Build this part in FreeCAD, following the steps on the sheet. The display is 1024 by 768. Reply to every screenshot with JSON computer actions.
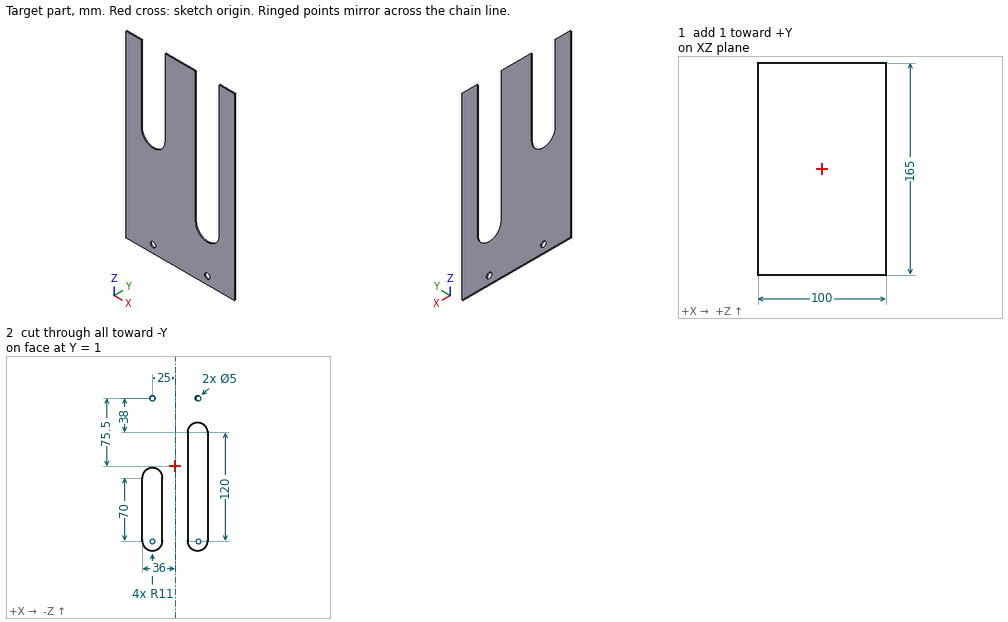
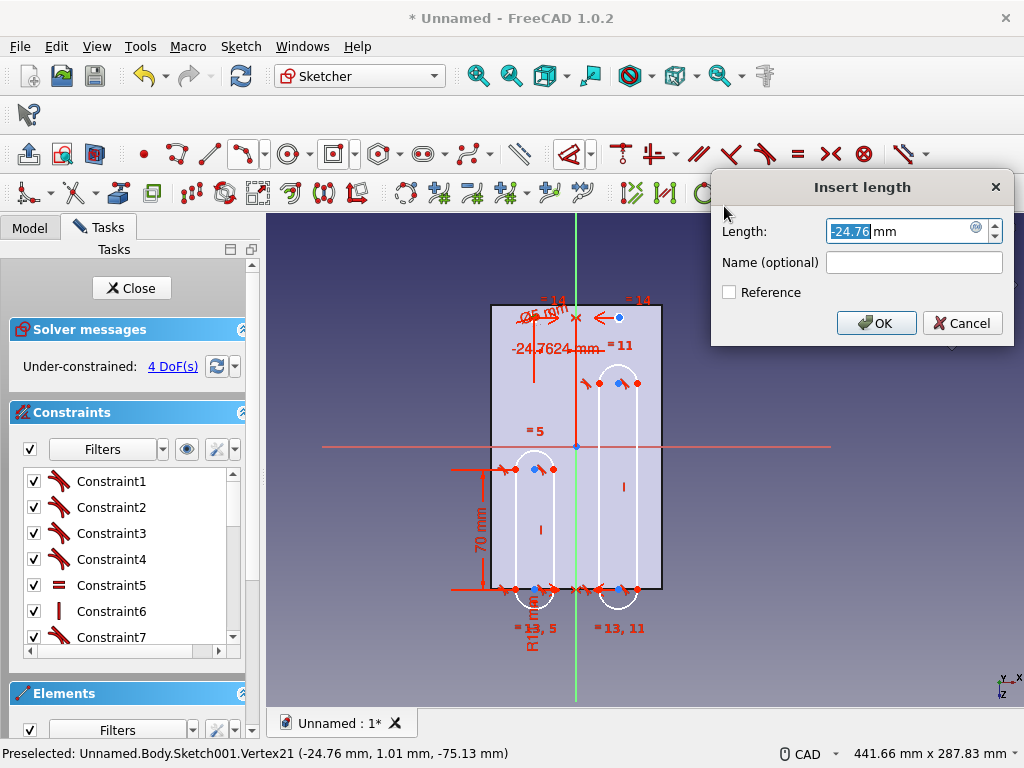
{"action": "type", "text": "-25"}
{"action": "key", "text": "Return"}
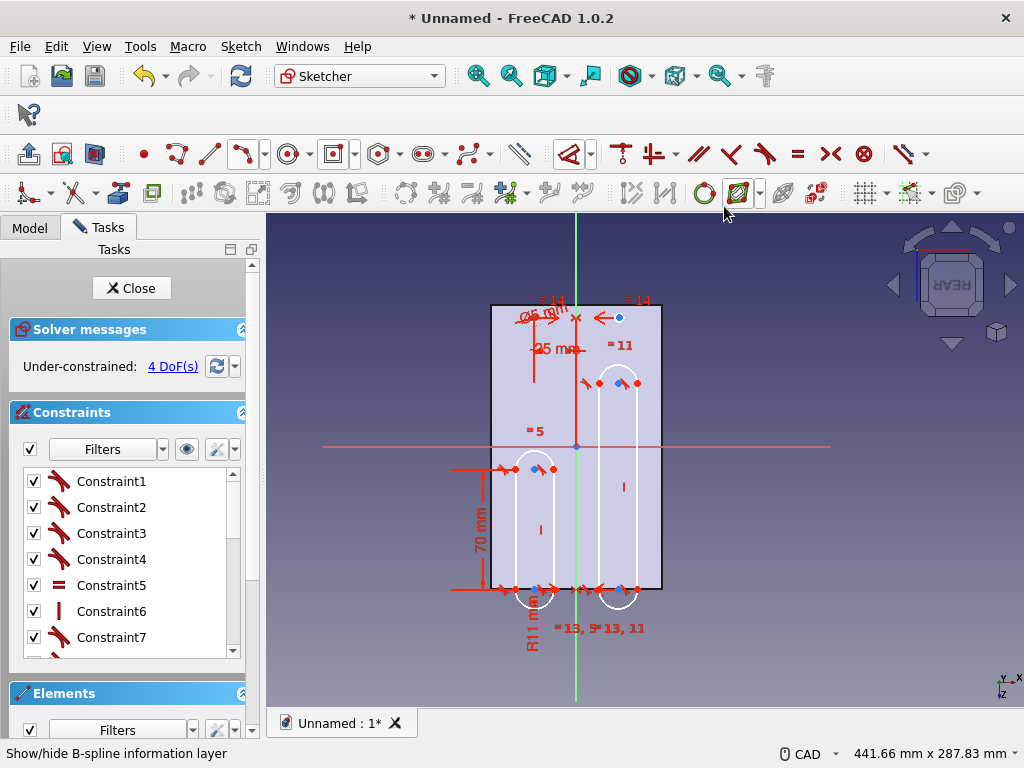
{"action": "left_click", "coordinate": [599, 528]}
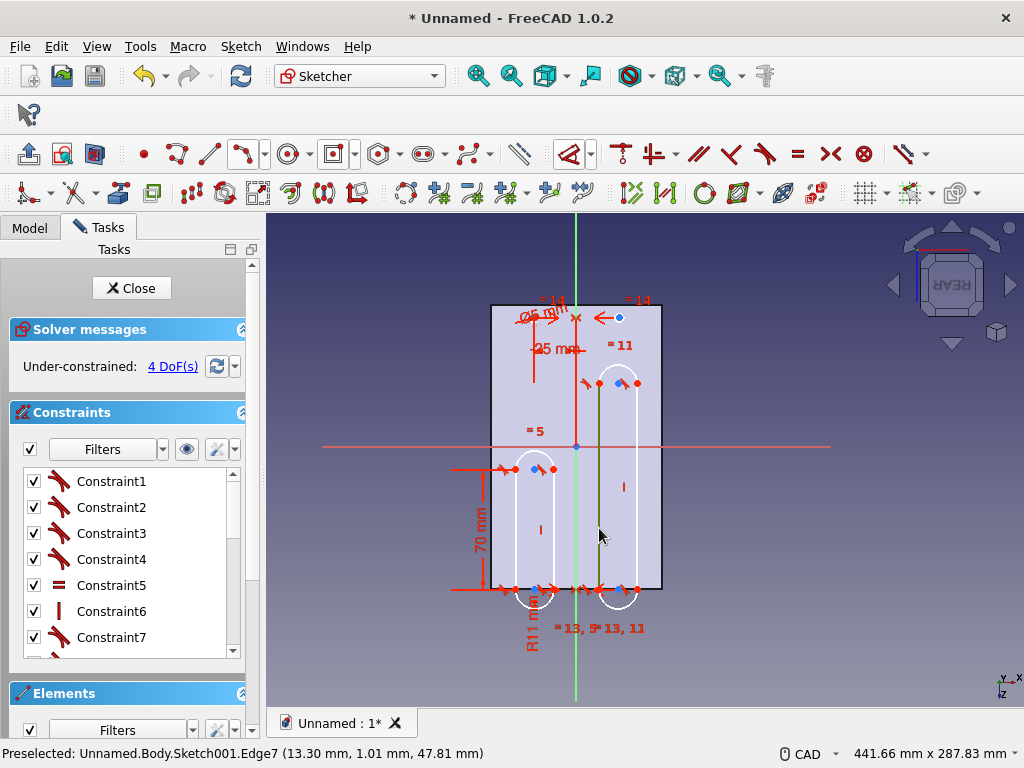
{"action": "left_click", "coordinate": [590, 154]}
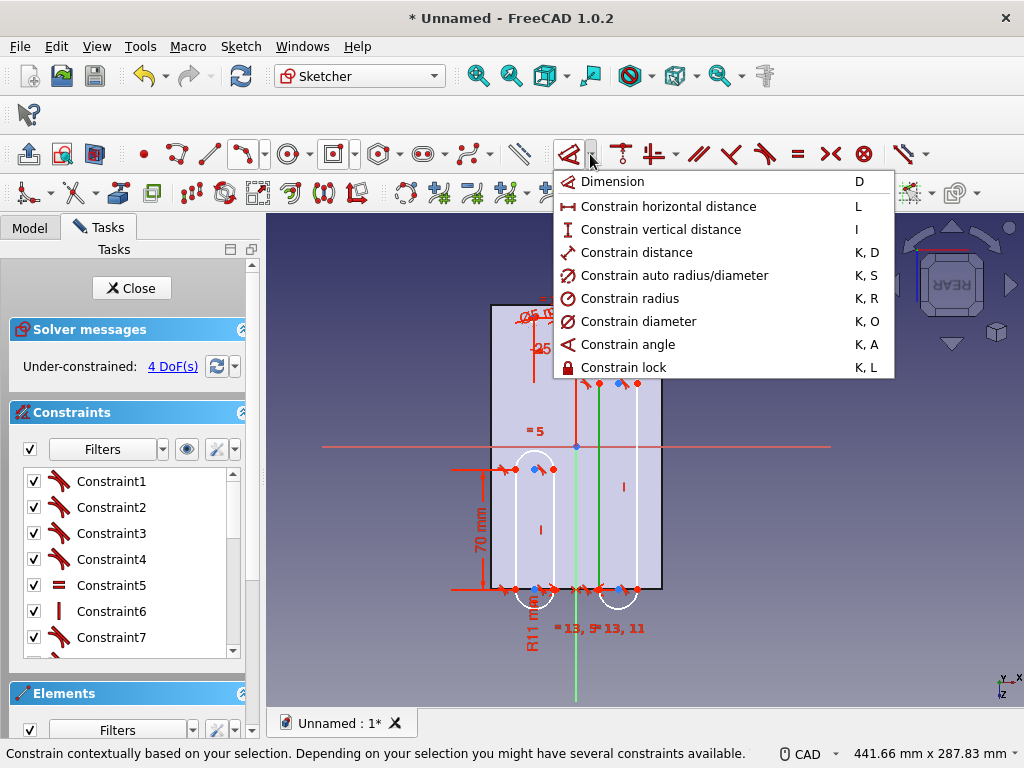
{"action": "left_click", "coordinate": [724, 230]}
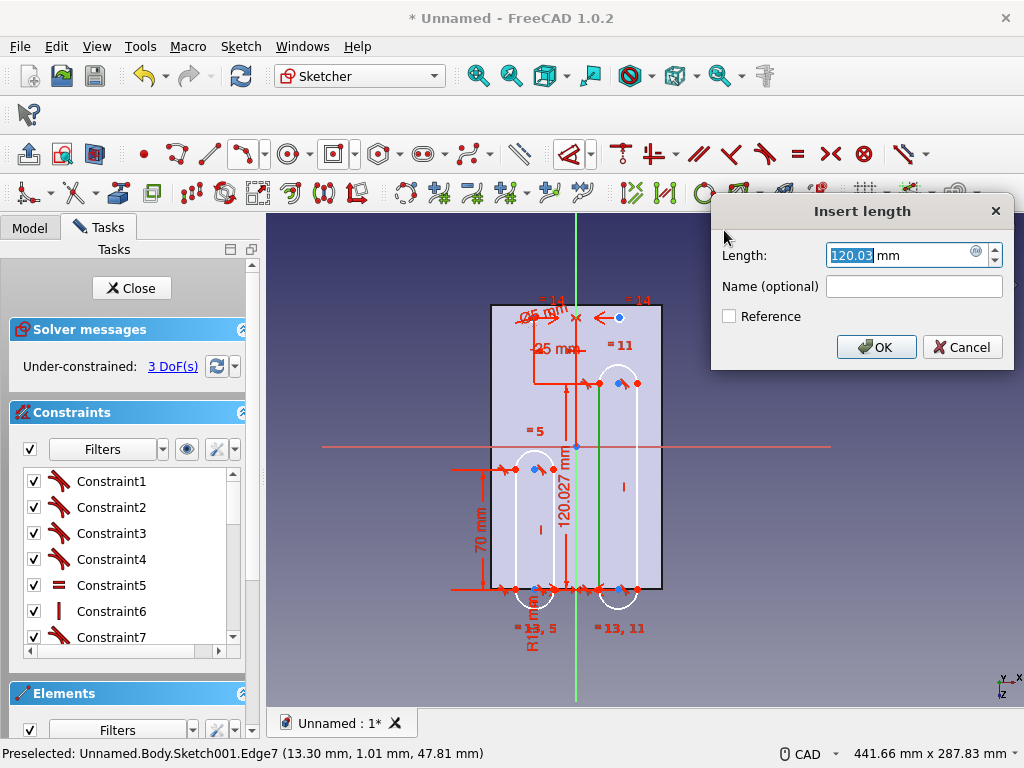
{"action": "type", "text": "120"}
{"action": "key", "text": "Return"}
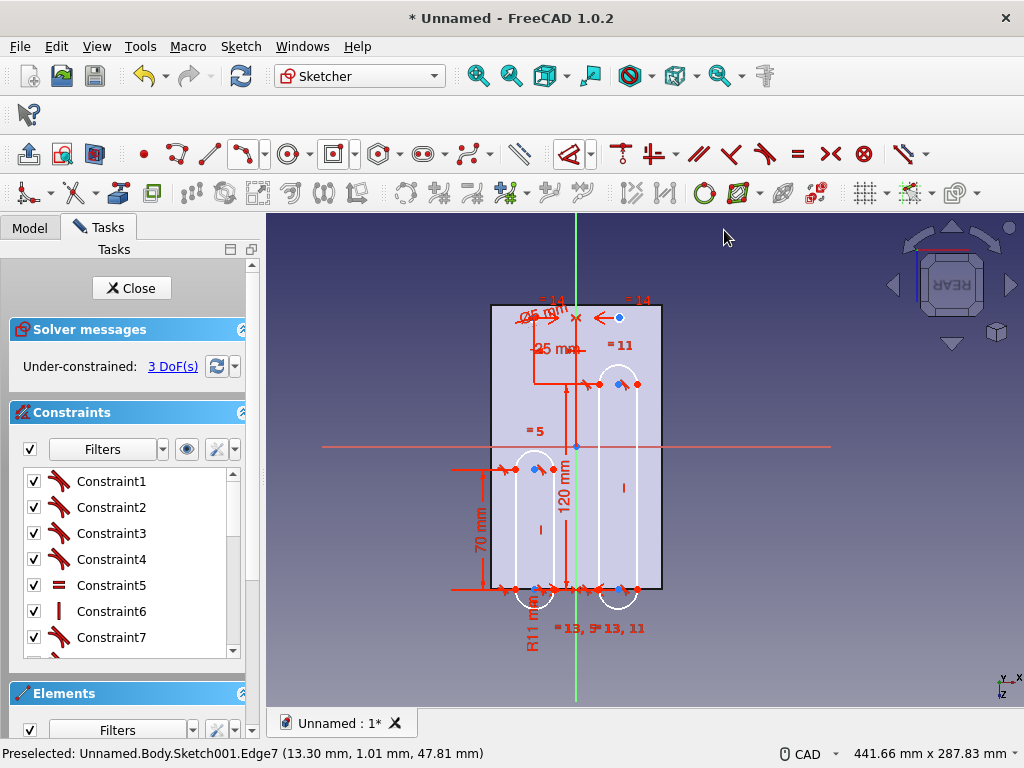
{"action": "left_click", "coordinate": [516, 590]}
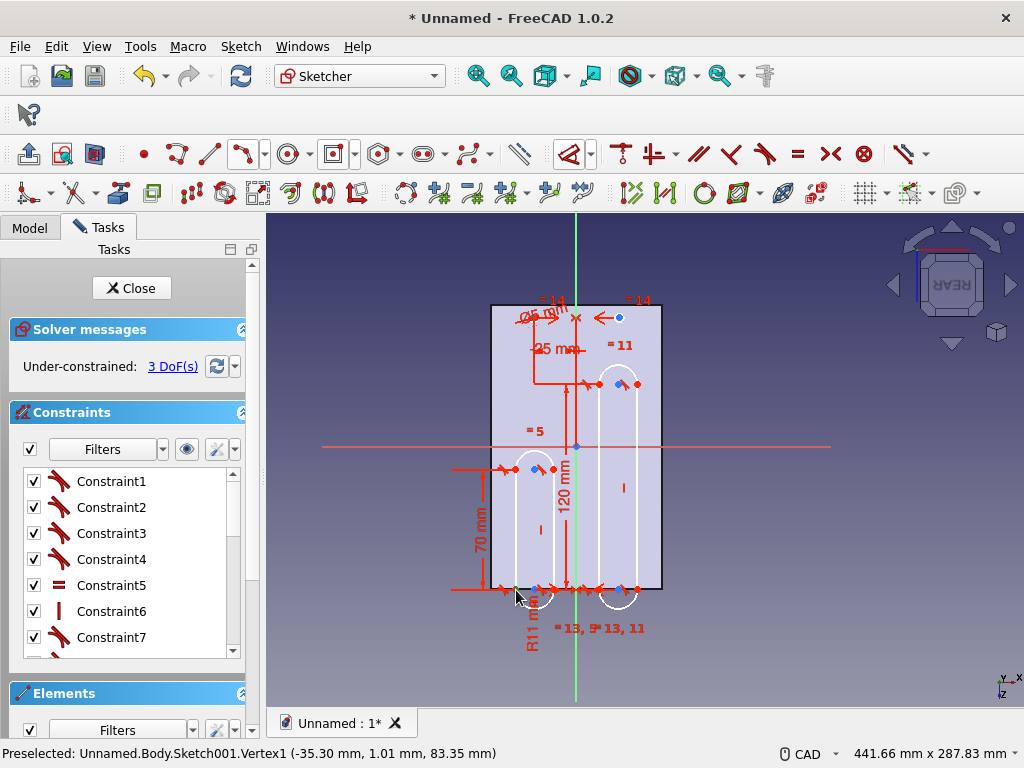
{"action": "key", "text": "l"}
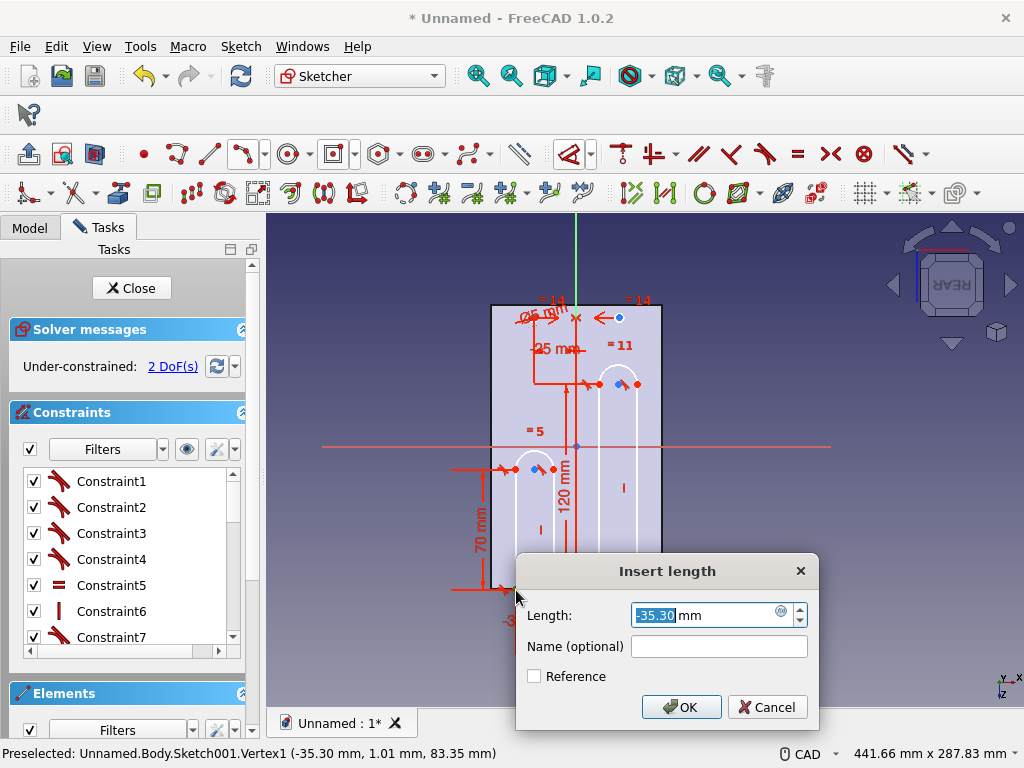
{"action": "type", "text": "-36"}
{"action": "key", "text": "Return"}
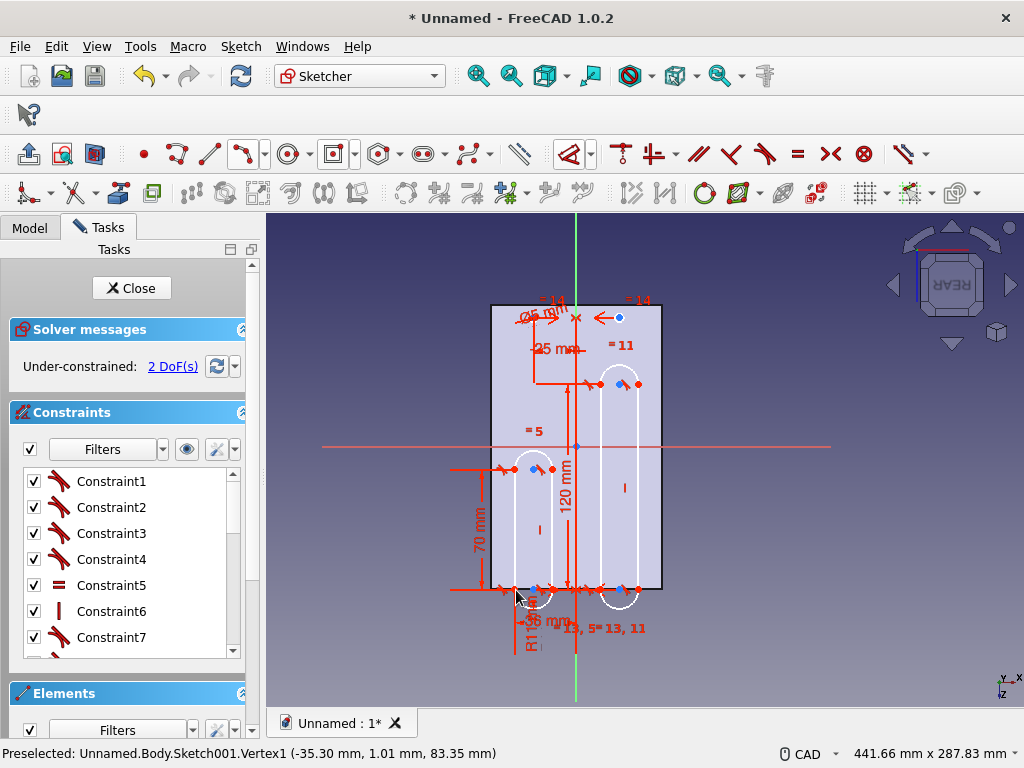
{"action": "left_click", "coordinate": [601, 384]}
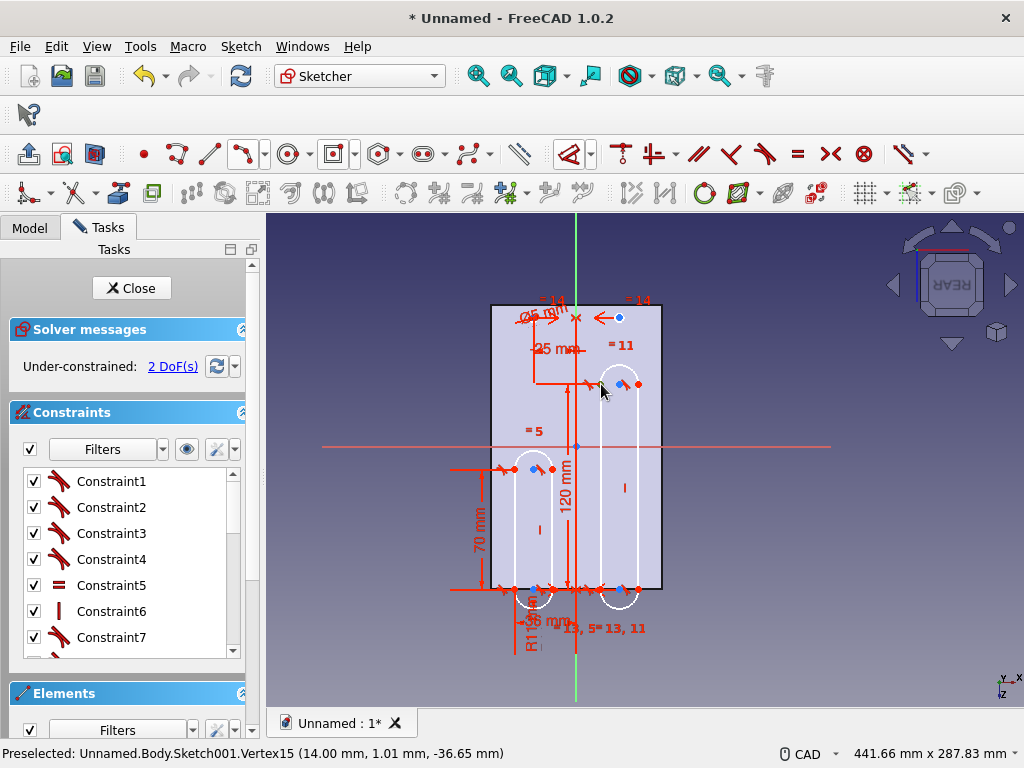
{"action": "left_click", "coordinate": [534, 318]}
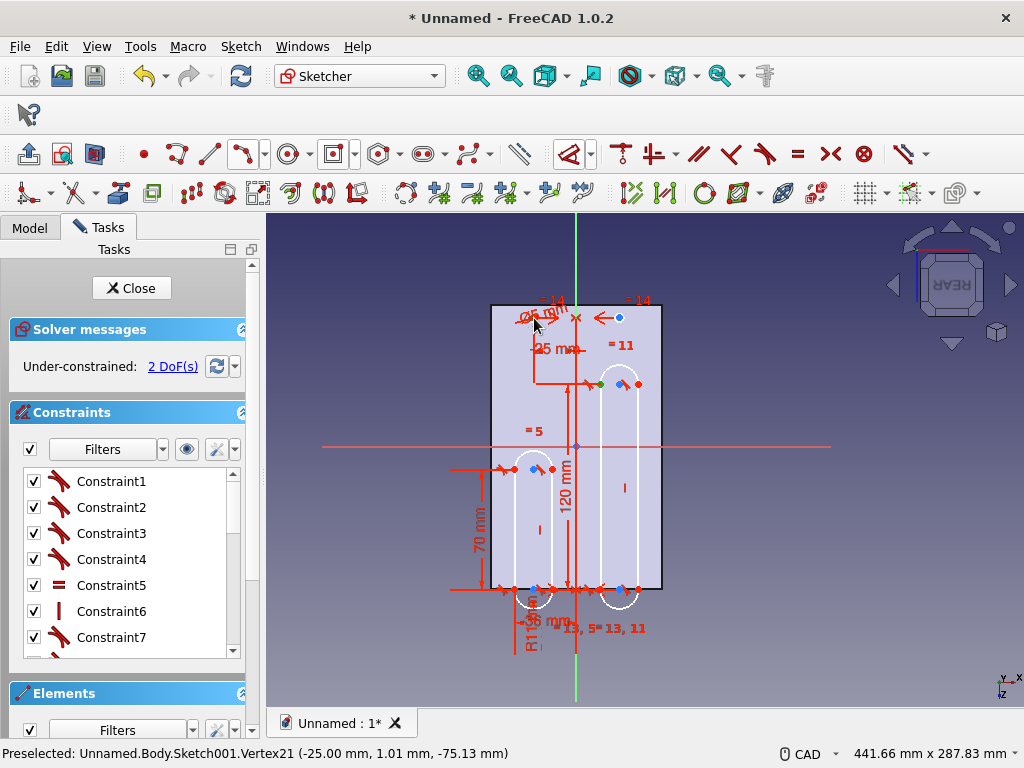
{"action": "left_click", "coordinate": [590, 154]}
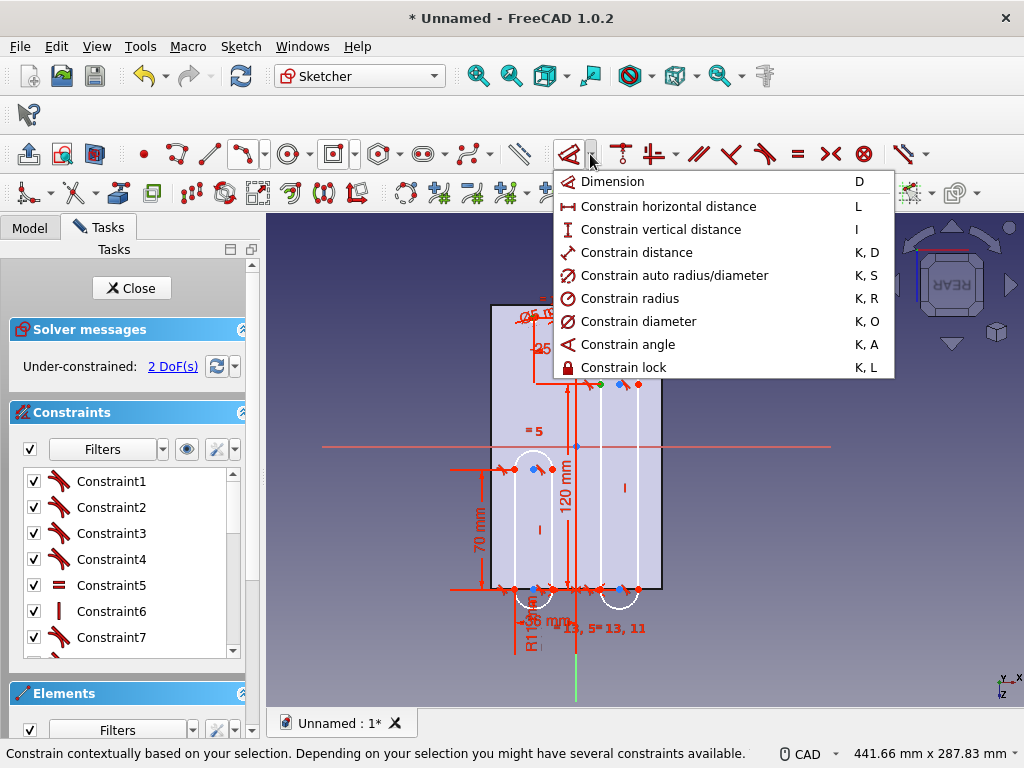
{"action": "left_click", "coordinate": [724, 230]}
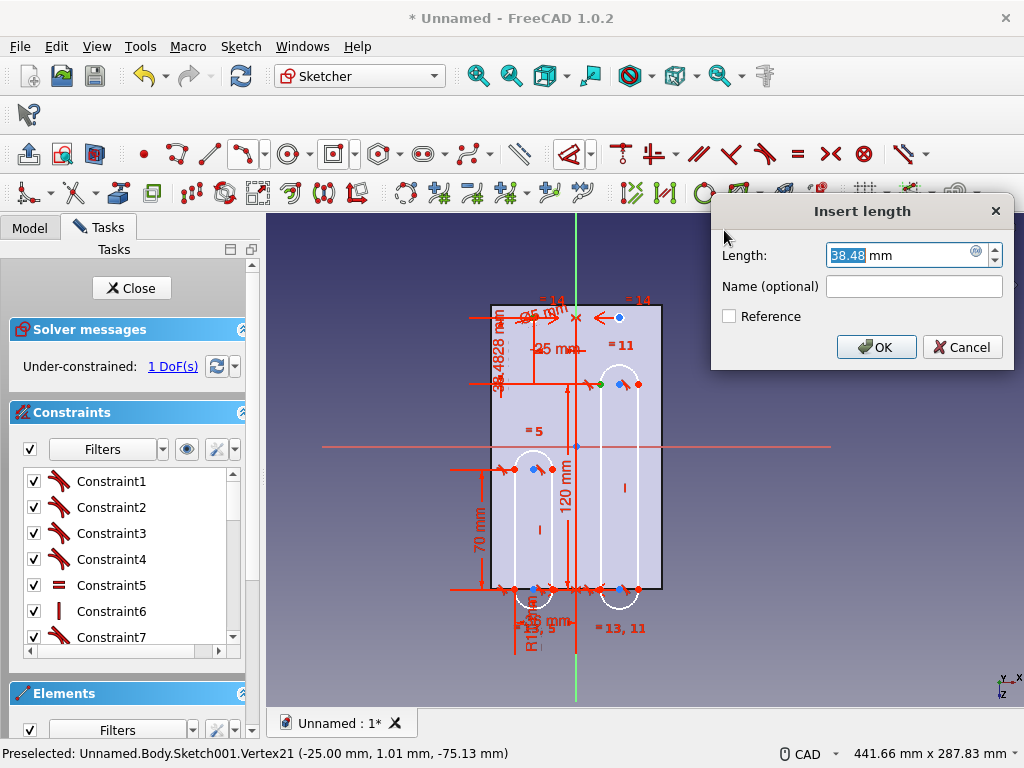
{"action": "type", "text": "38"}
{"action": "key", "text": "Return"}